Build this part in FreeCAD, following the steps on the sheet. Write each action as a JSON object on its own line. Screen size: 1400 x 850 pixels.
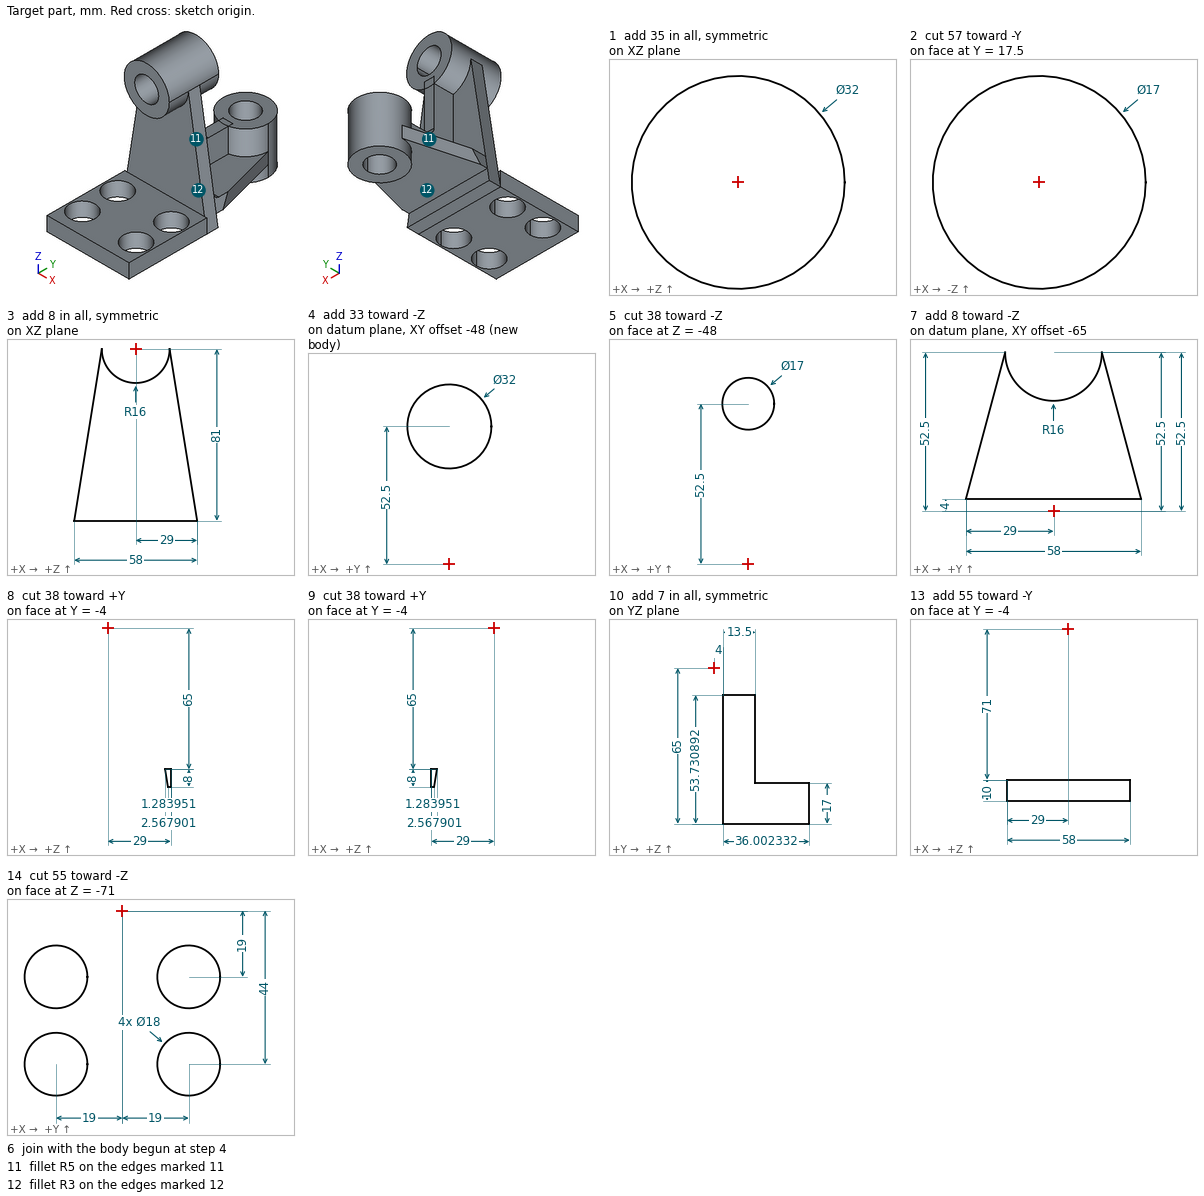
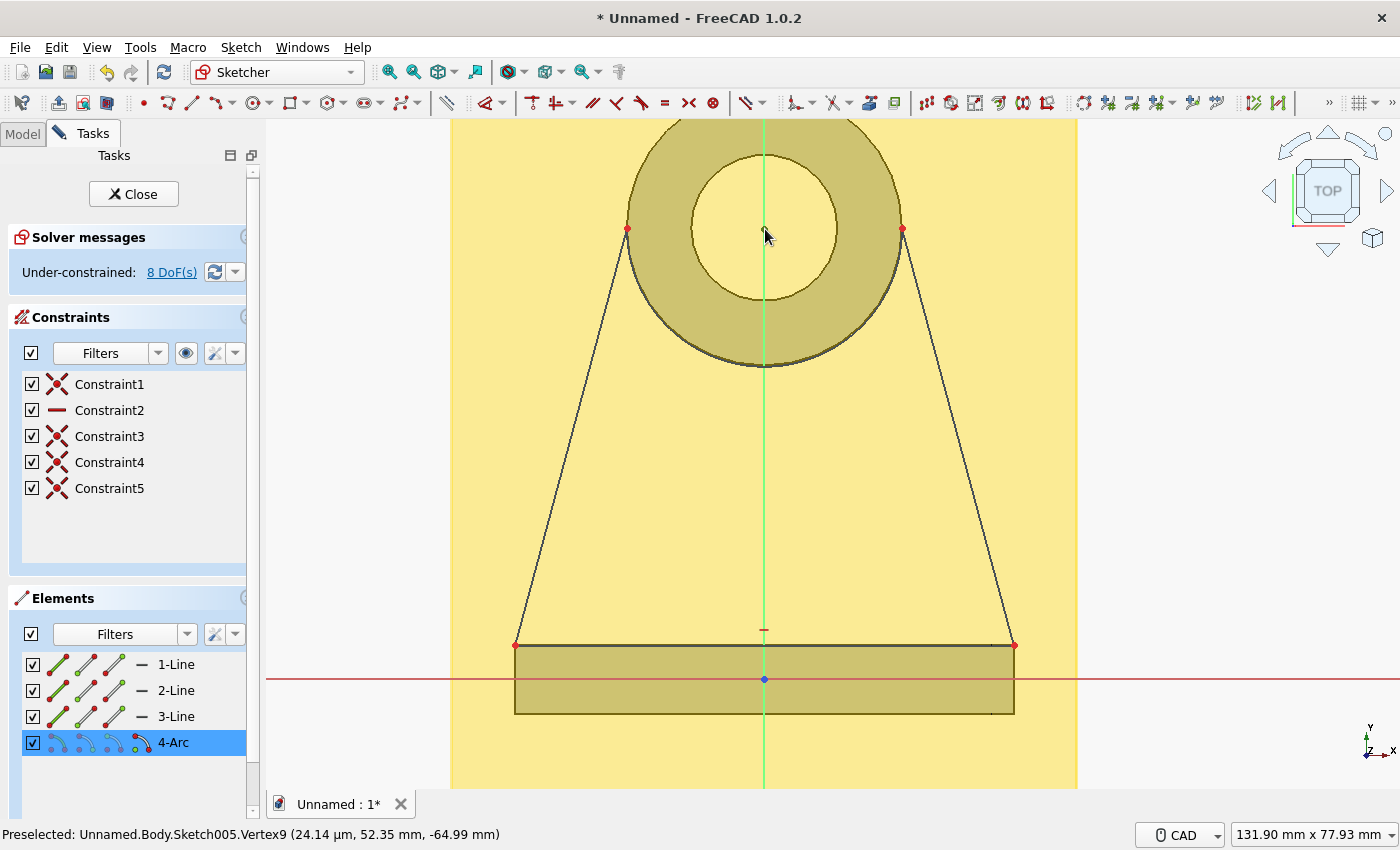
{"action": "left_click", "coordinate": [764, 717]}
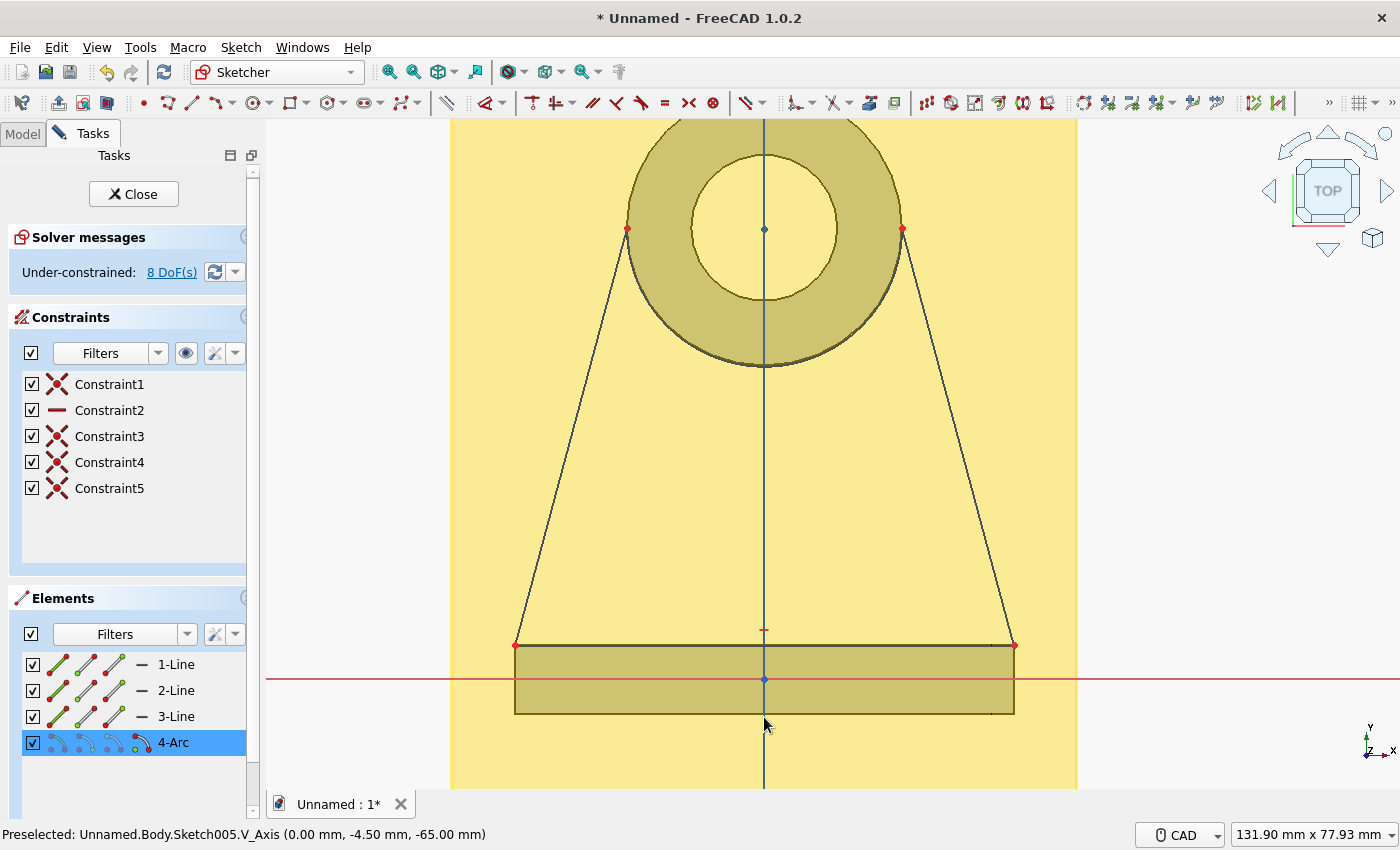
{"action": "key", "text": "c"}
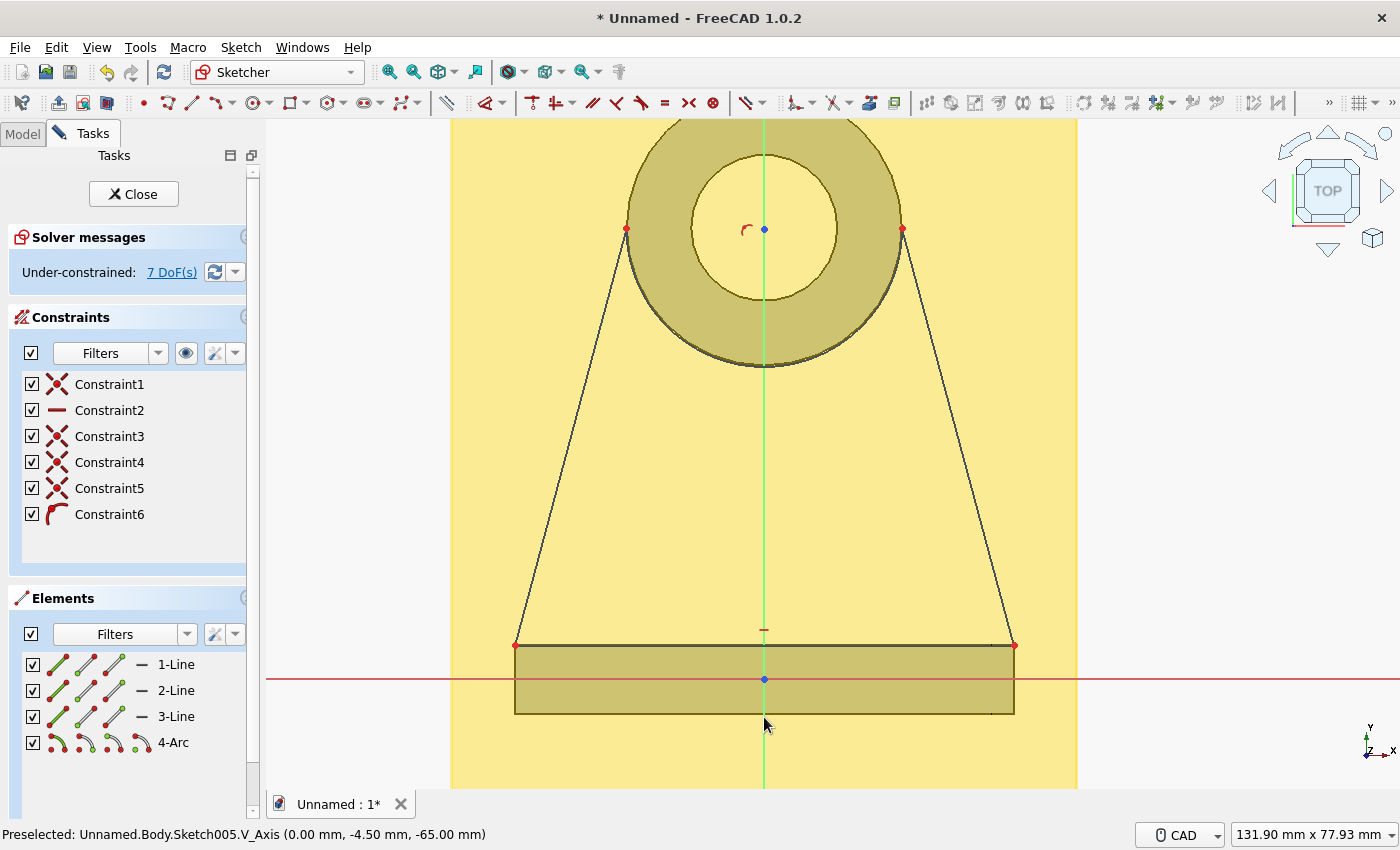
{"action": "left_click", "coordinate": [486, 104]}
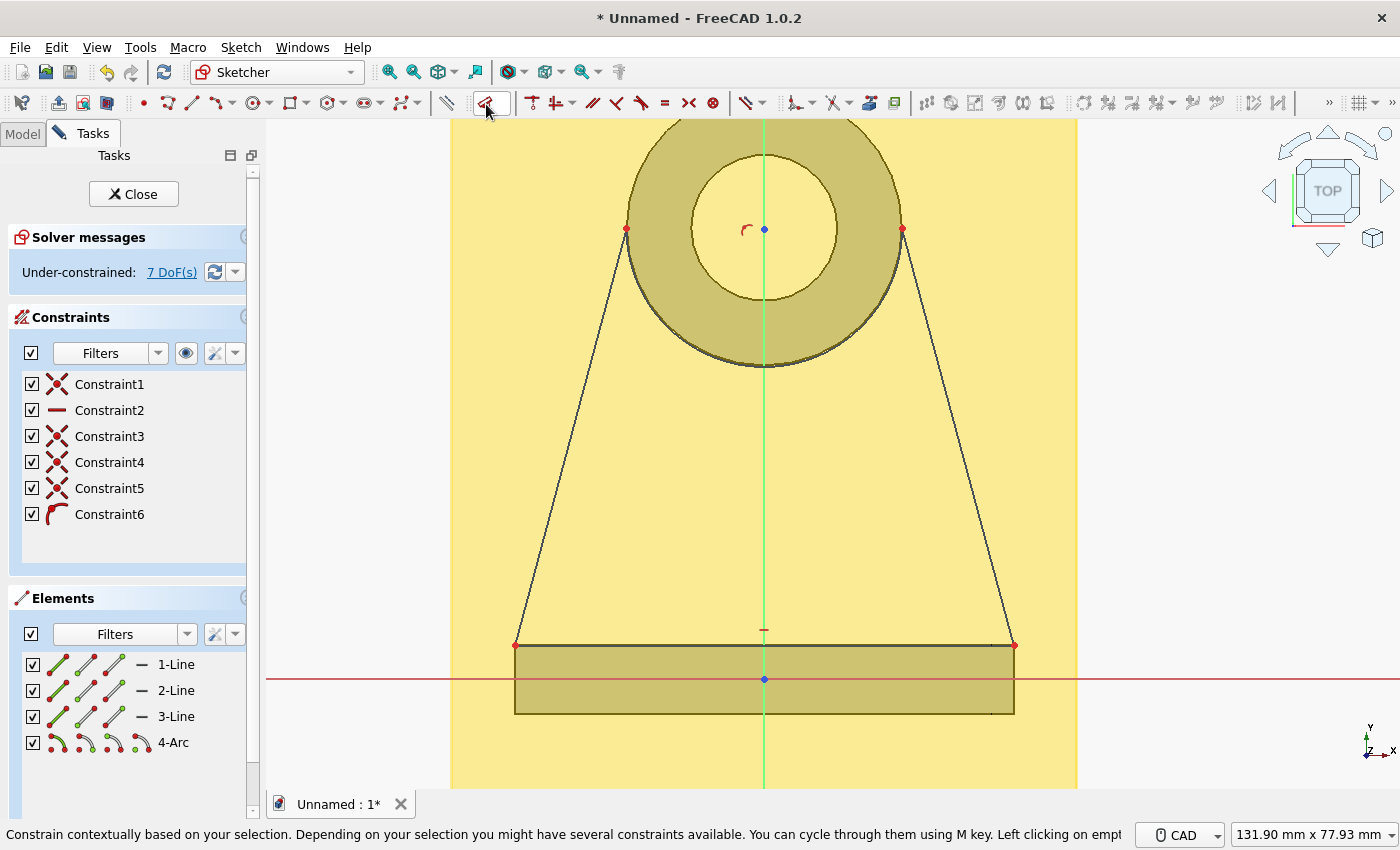
{"action": "left_click", "coordinate": [683, 341]}
{"action": "left_click", "coordinate": [664, 367]}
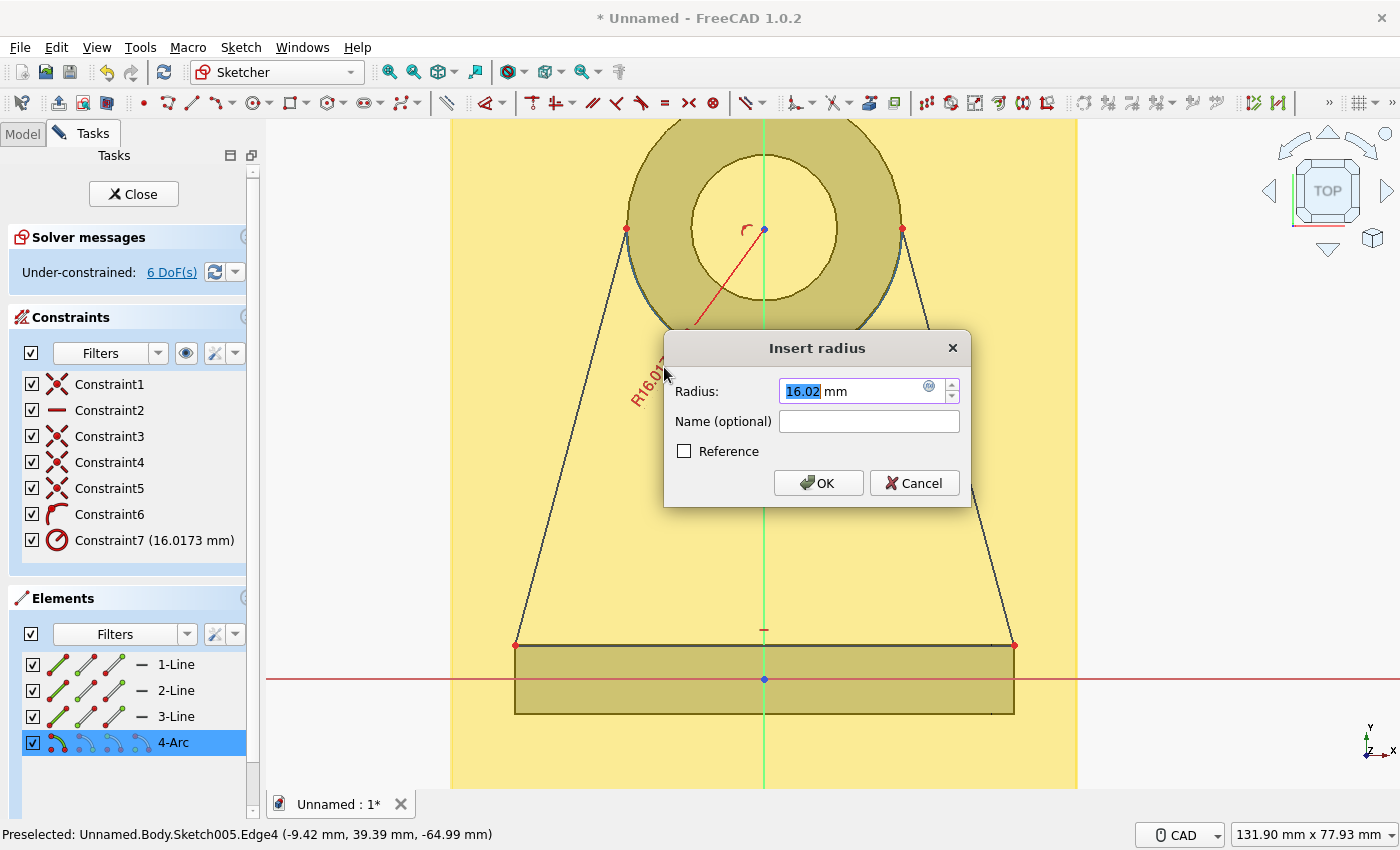
{"action": "type", "text": "16"}
{"action": "key", "text": "Return"}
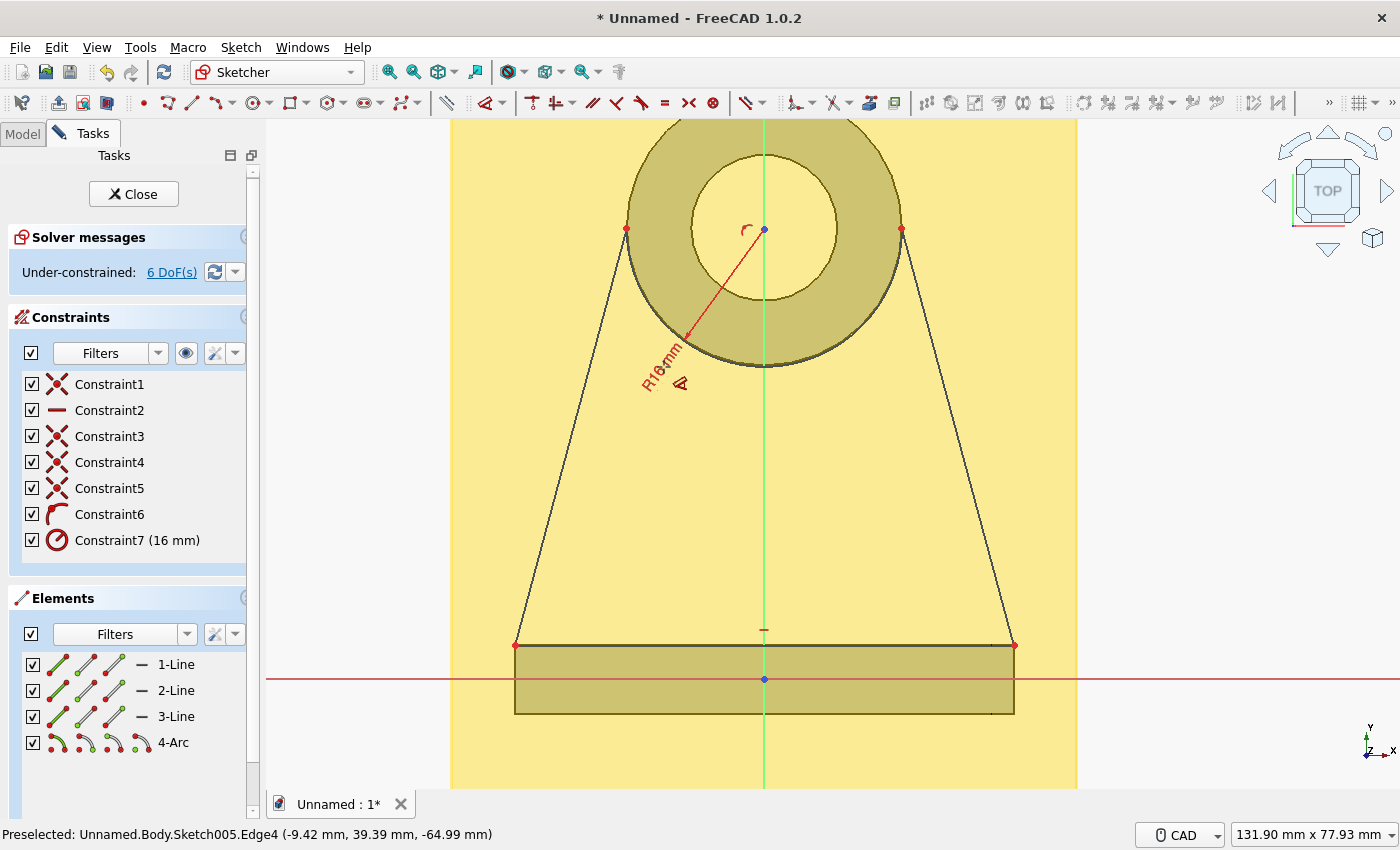
{"action": "left_click", "coordinate": [665, 646]}
{"action": "left_click", "coordinate": [650, 612]}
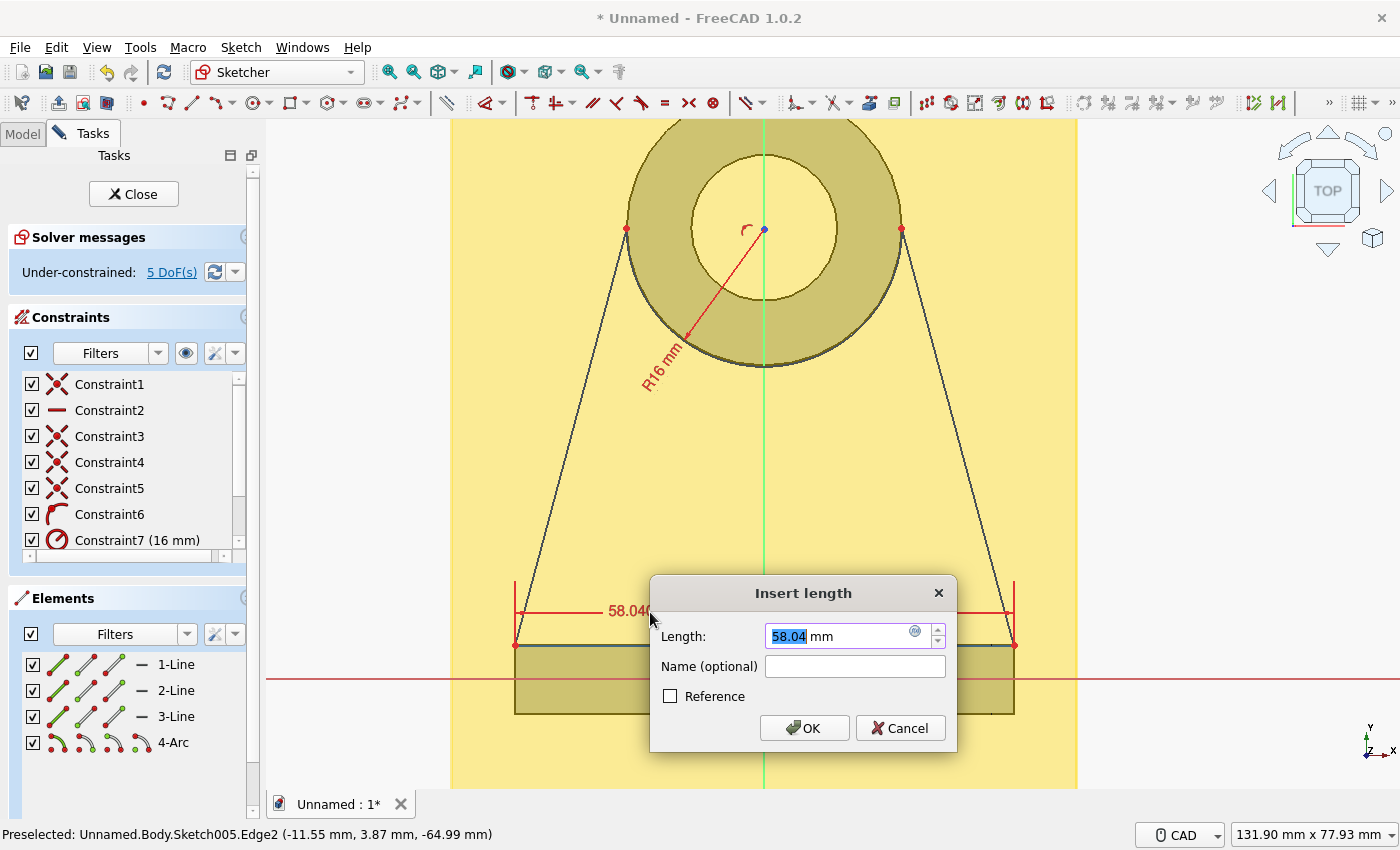
{"action": "type", "text": "58"}
{"action": "key", "text": "Return"}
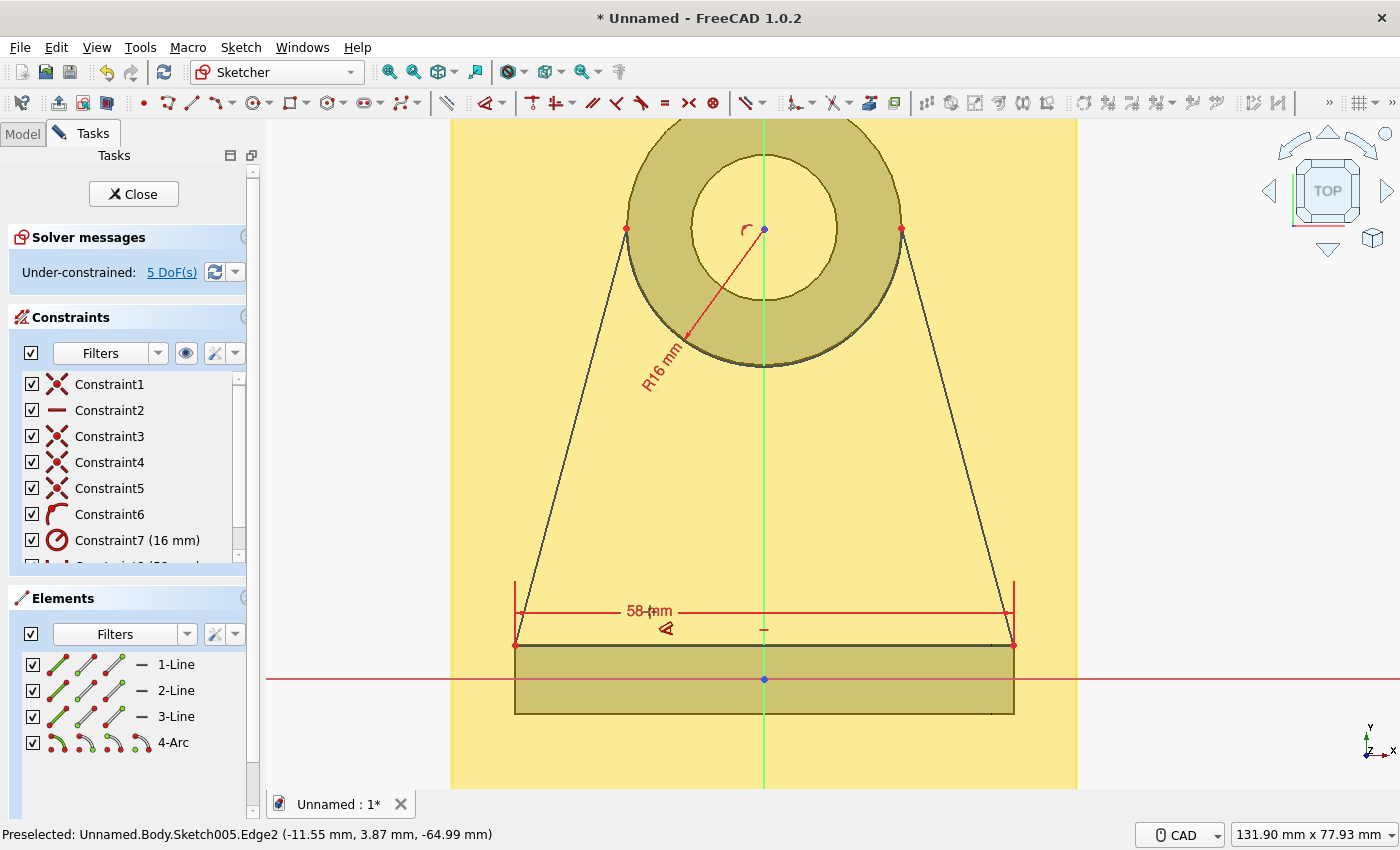
{"action": "left_click", "coordinate": [515, 646]}
{"action": "left_click", "coordinate": [481, 663]}